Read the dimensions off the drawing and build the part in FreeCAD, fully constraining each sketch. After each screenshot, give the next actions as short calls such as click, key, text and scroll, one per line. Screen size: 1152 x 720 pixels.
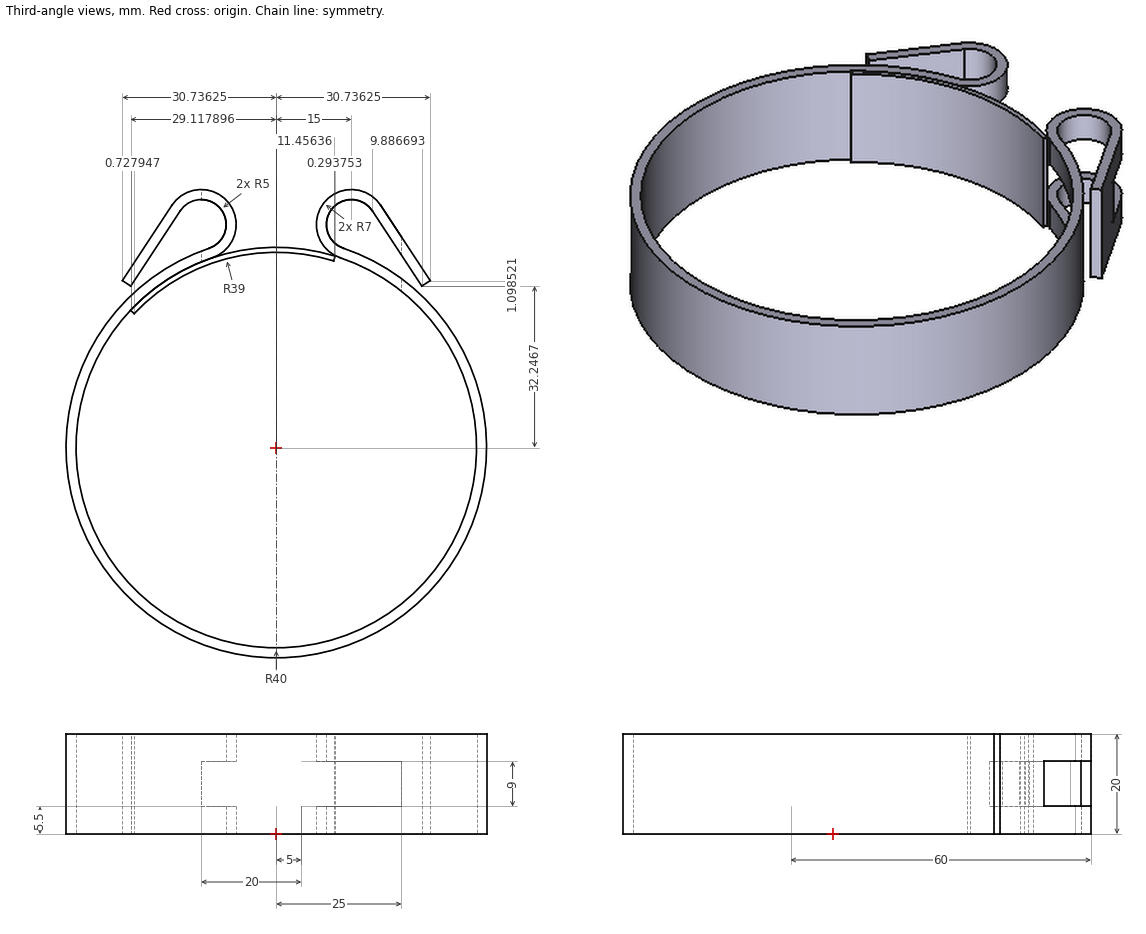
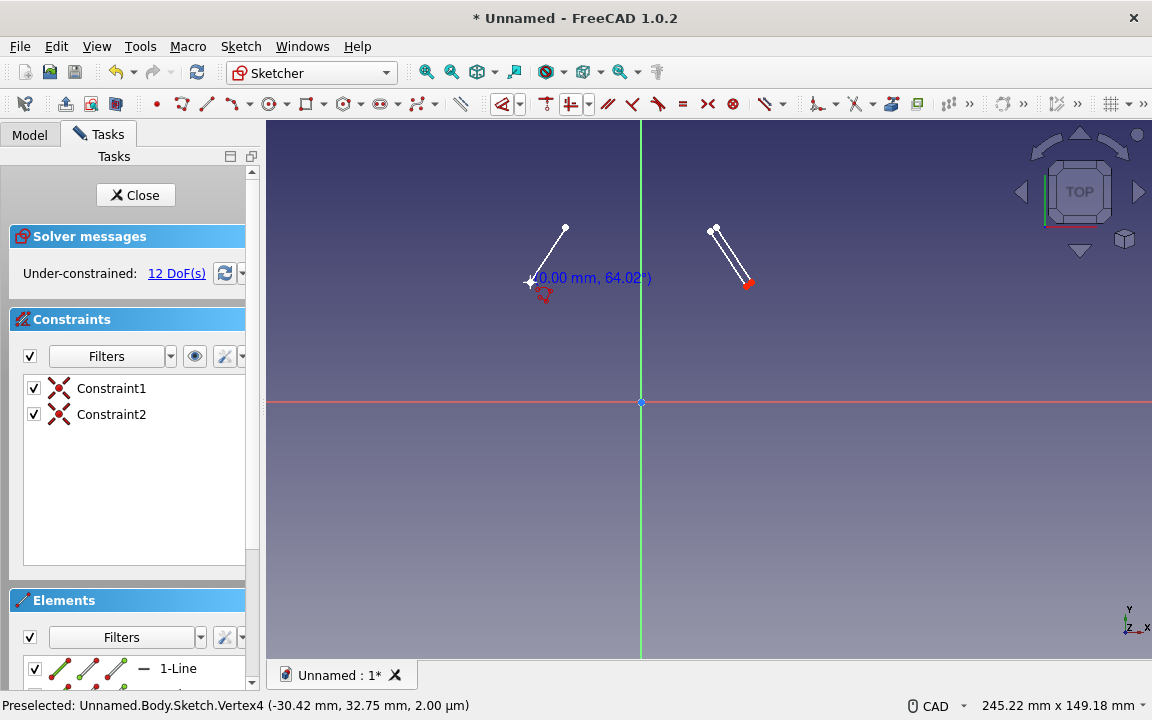
scroll(536, 286, up, 4)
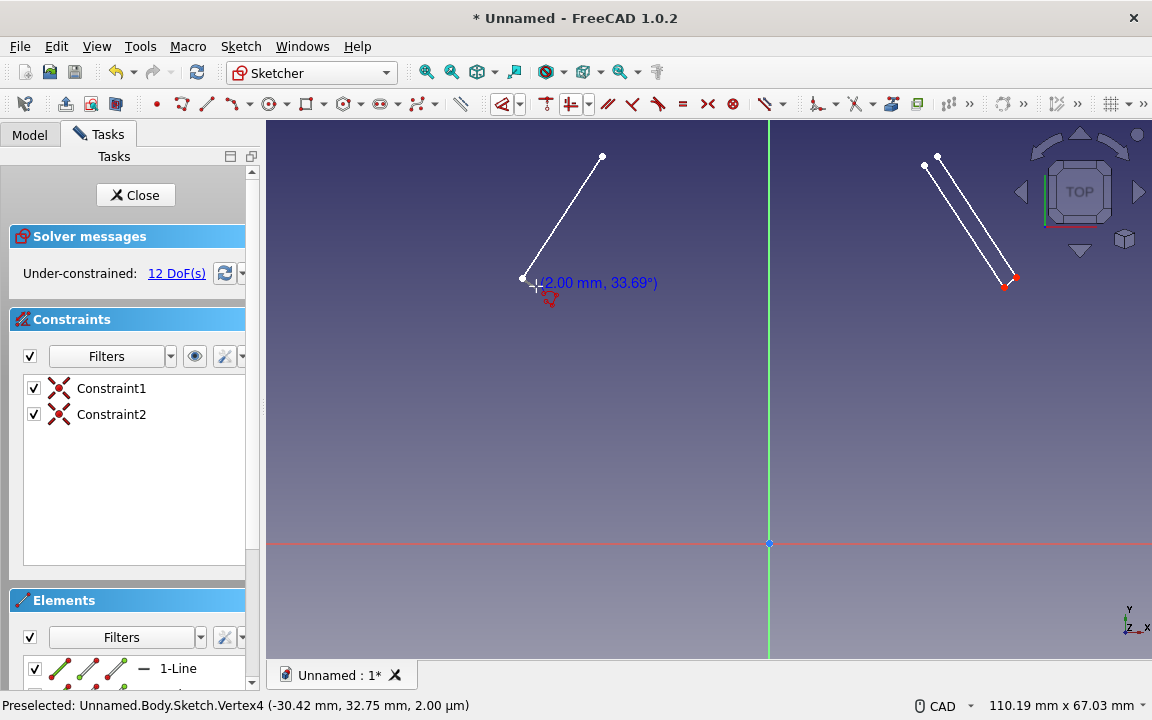
click(536, 285)
click(615, 164)
right_click(615, 164)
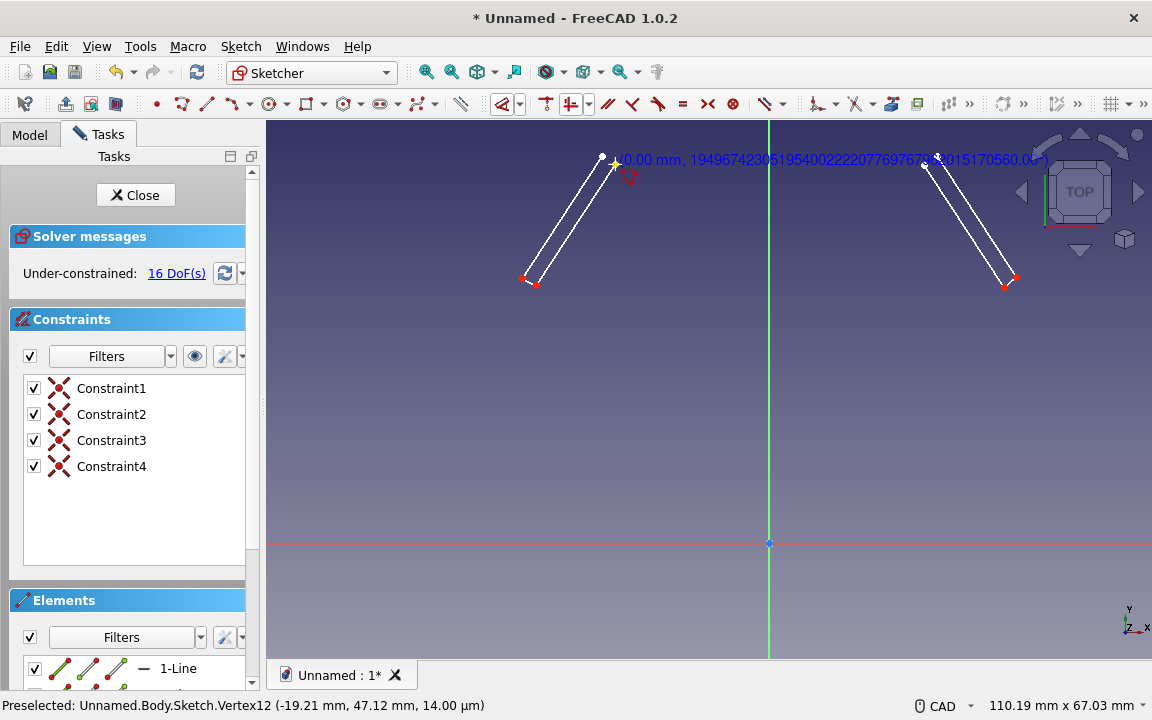
key(g)
key(3)
key(a)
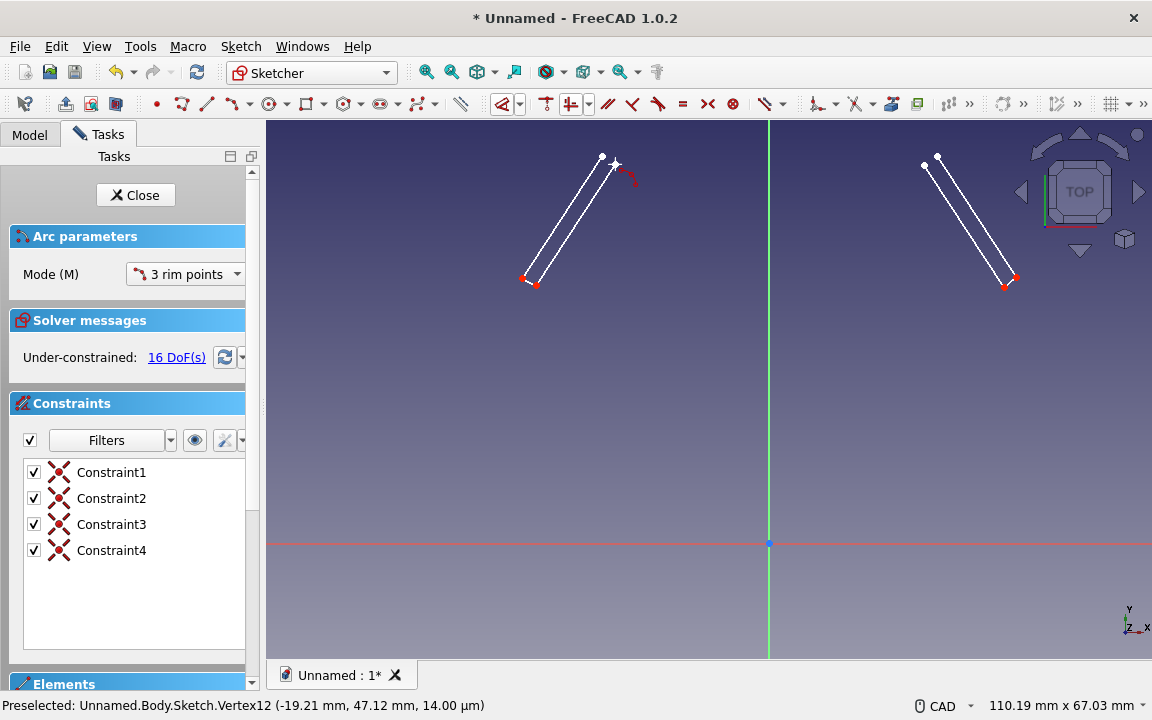
click(937, 156)
click(872, 239)
click(846, 151)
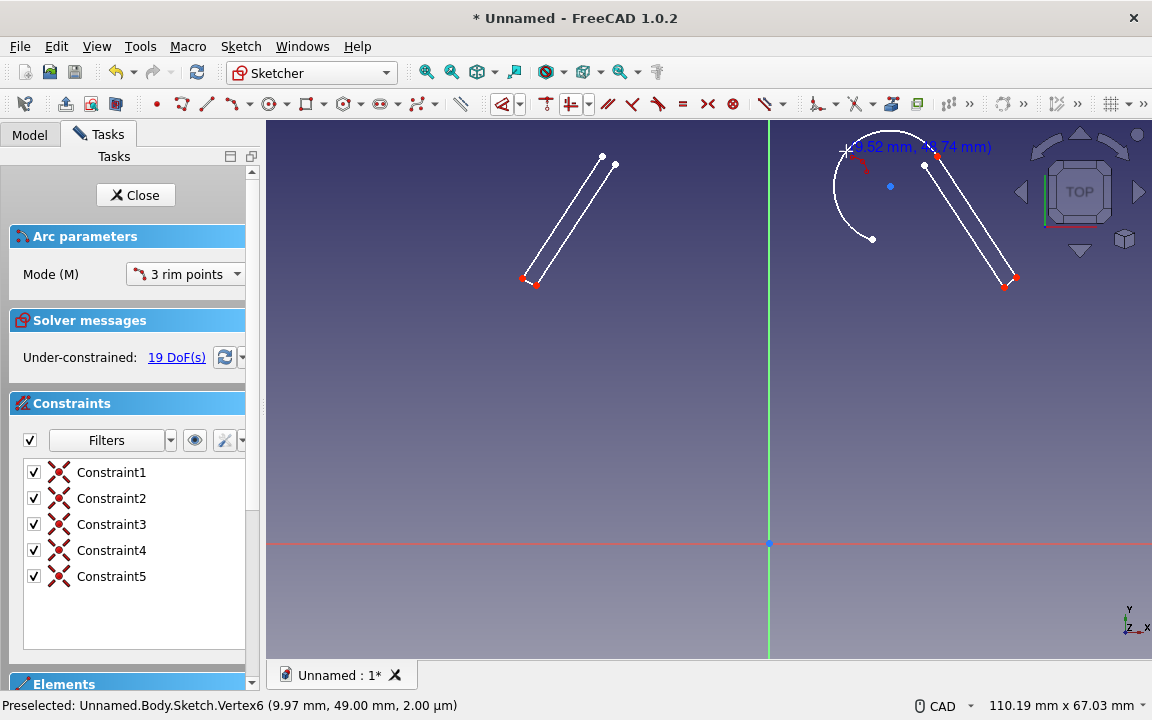
click(872, 240)
click(667, 239)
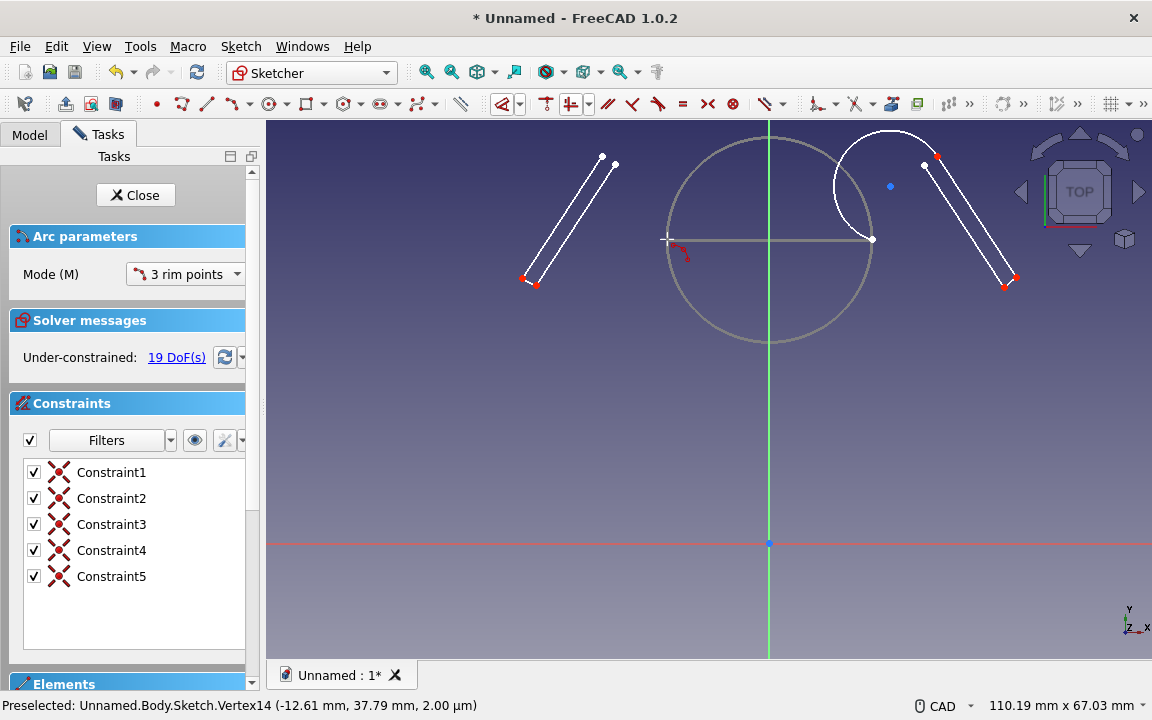
scroll(535, 286, down, 4)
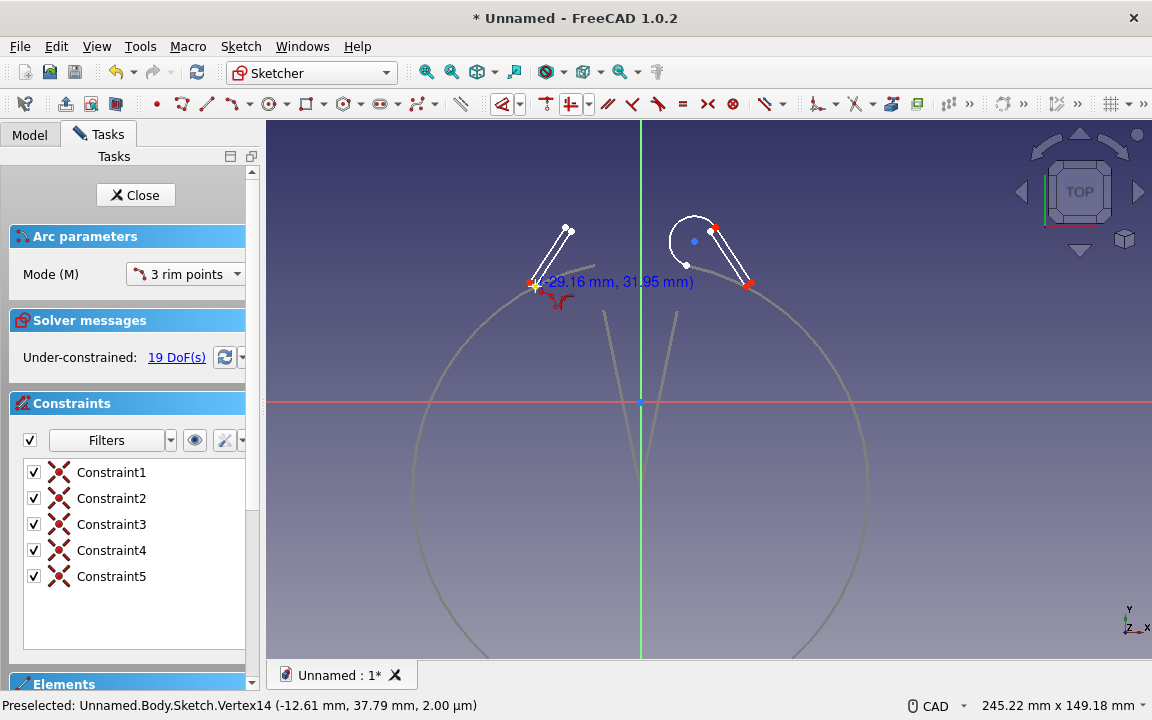
click(563, 524)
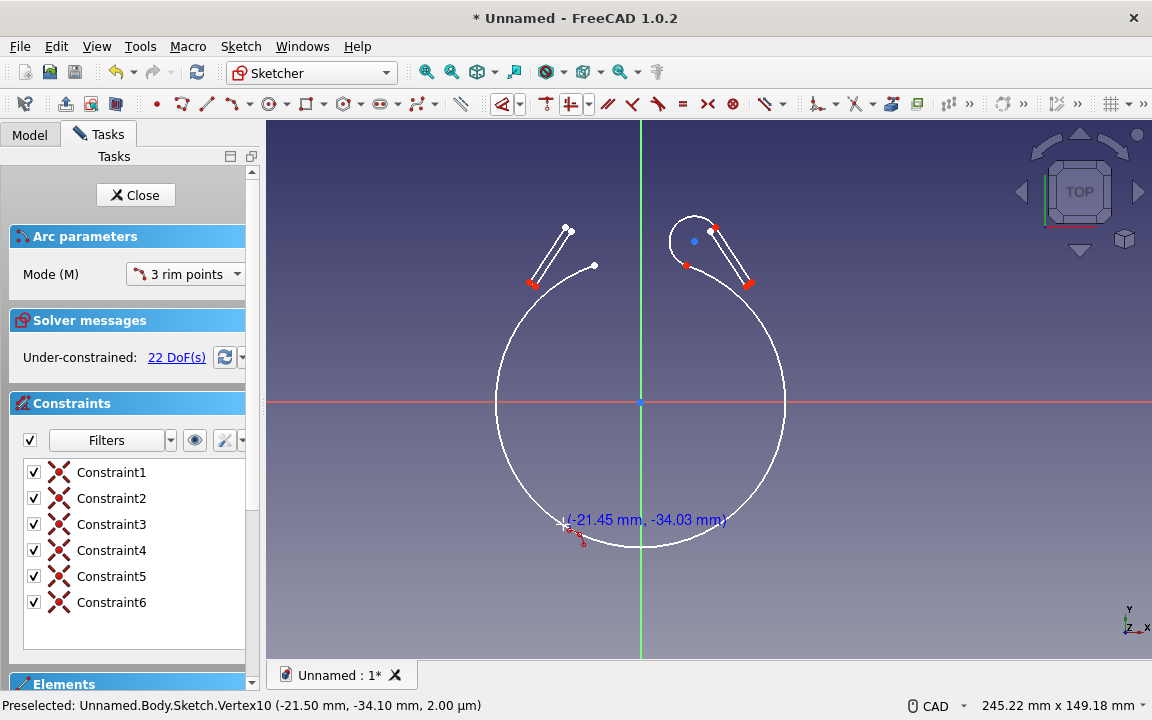
click(594, 266)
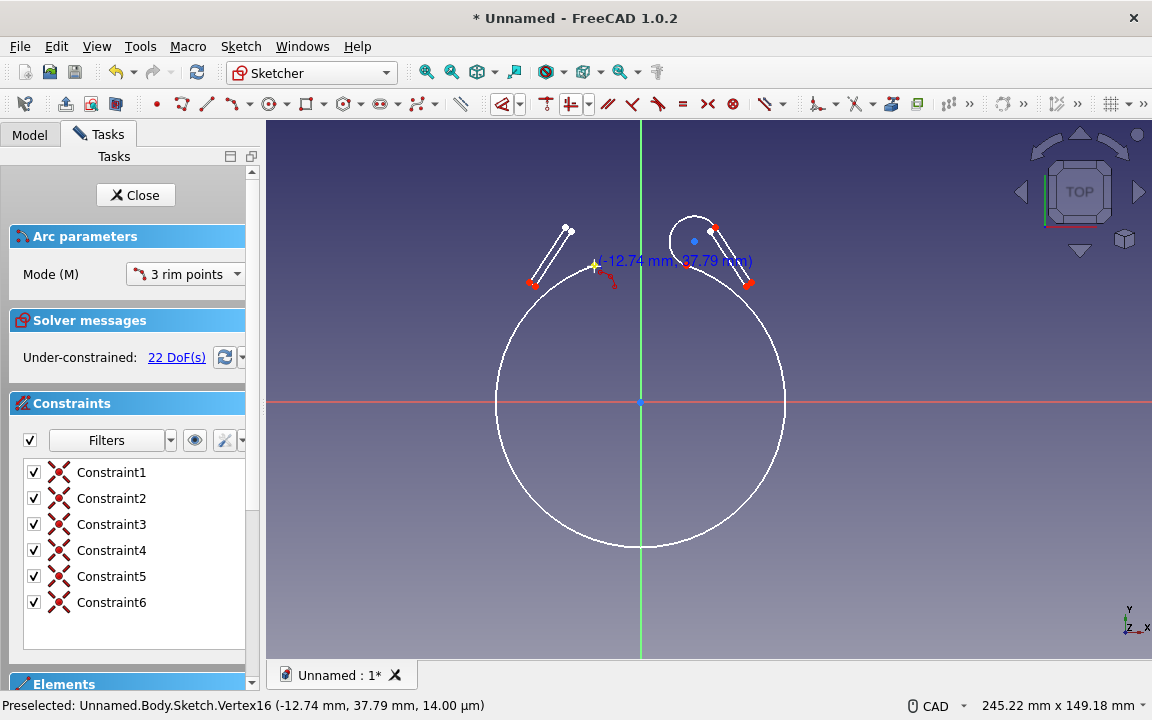
scroll(565, 227, up, 4)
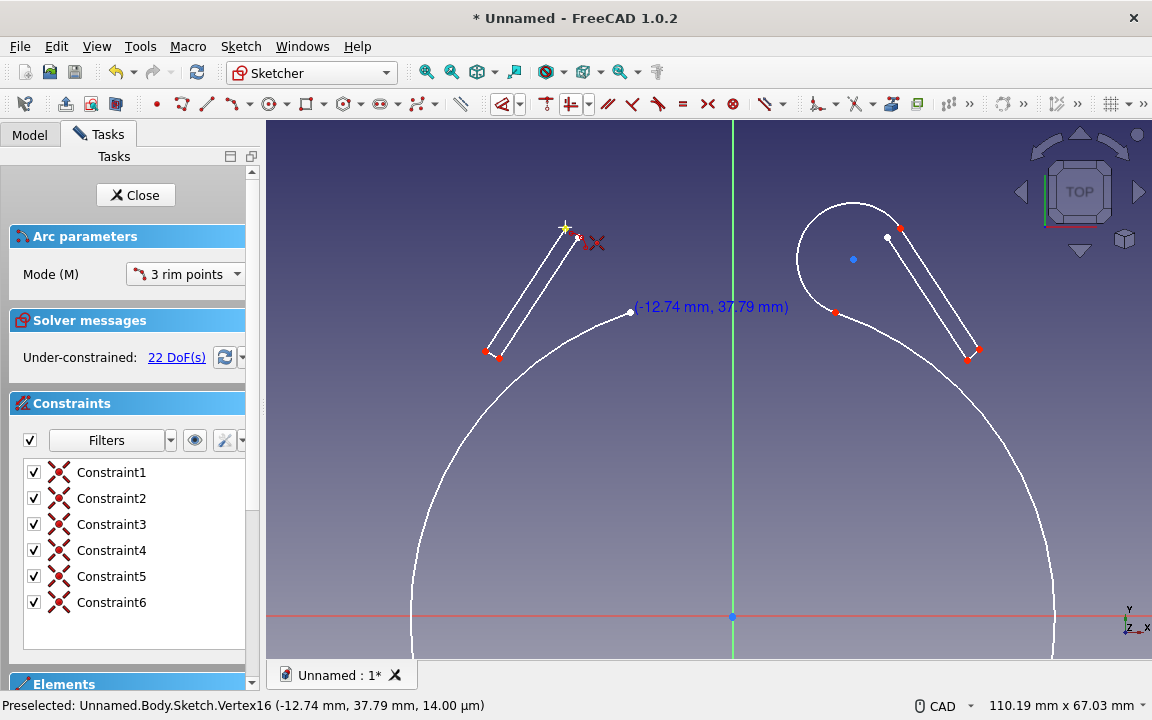
click(565, 229)
click(657, 224)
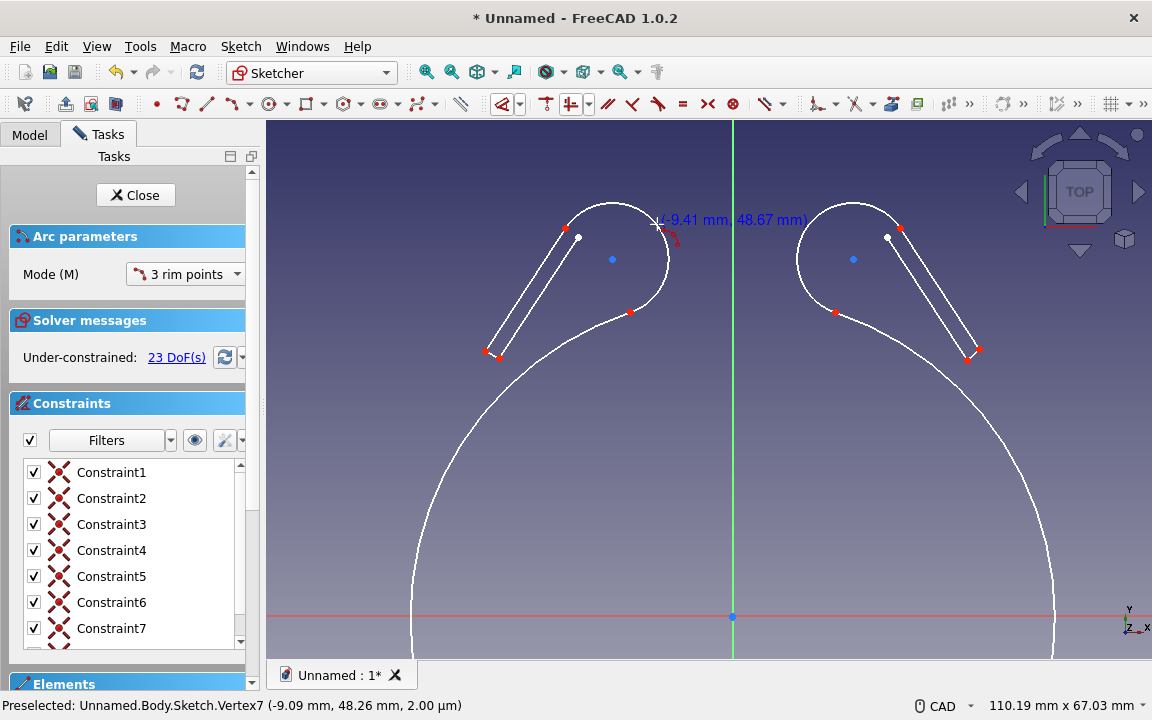
click(578, 237)
click(625, 296)
click(652, 262)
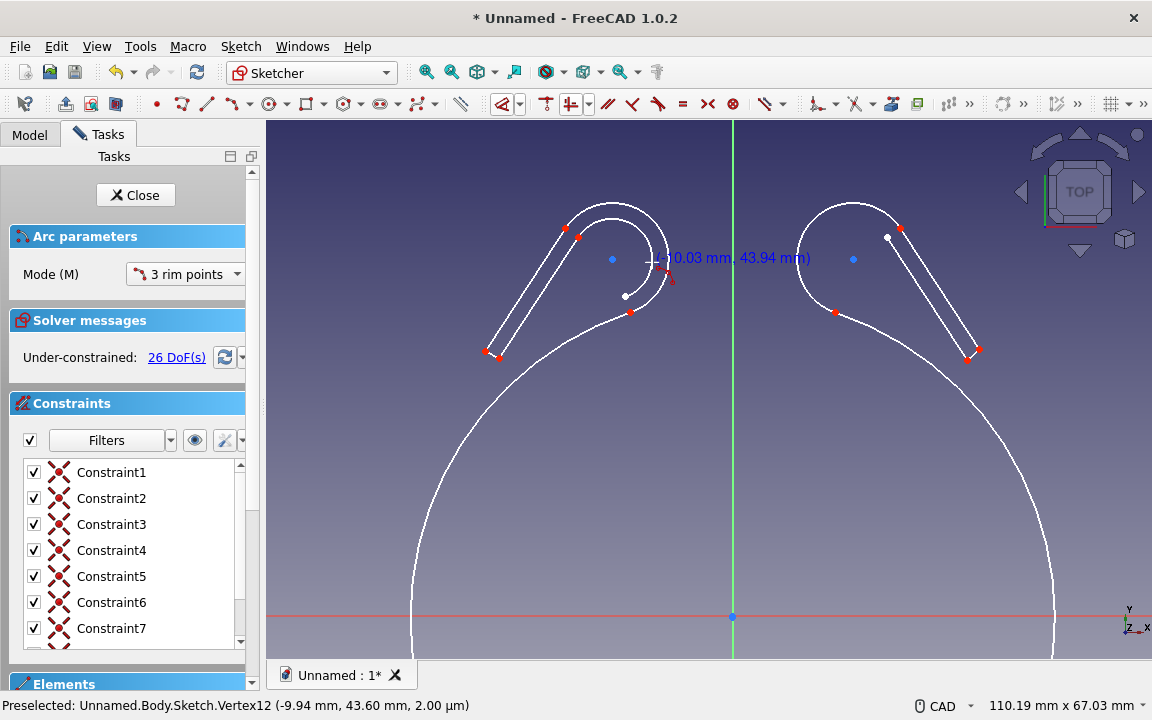
click(625, 297)
click(840, 296)